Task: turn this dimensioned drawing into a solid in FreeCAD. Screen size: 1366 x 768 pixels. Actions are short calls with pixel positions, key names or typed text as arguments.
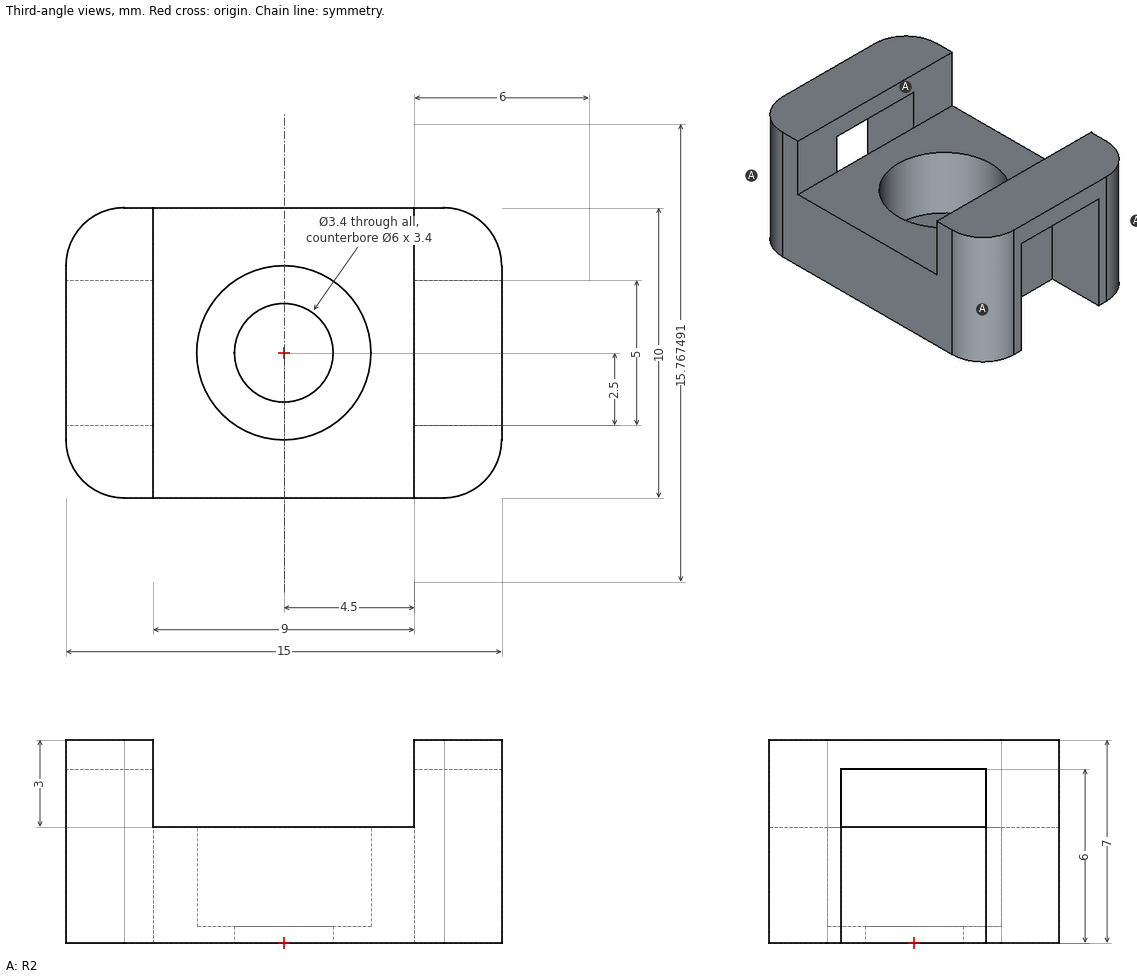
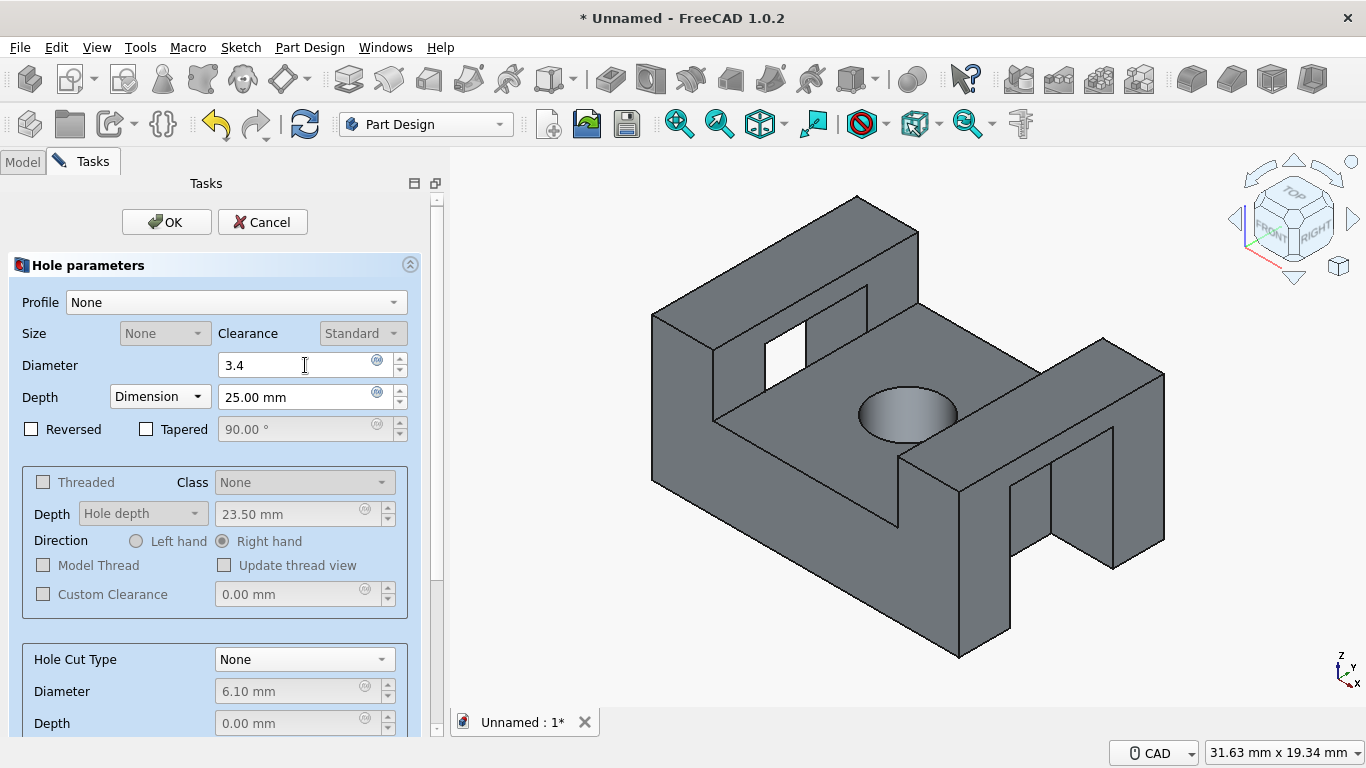
click(161, 396)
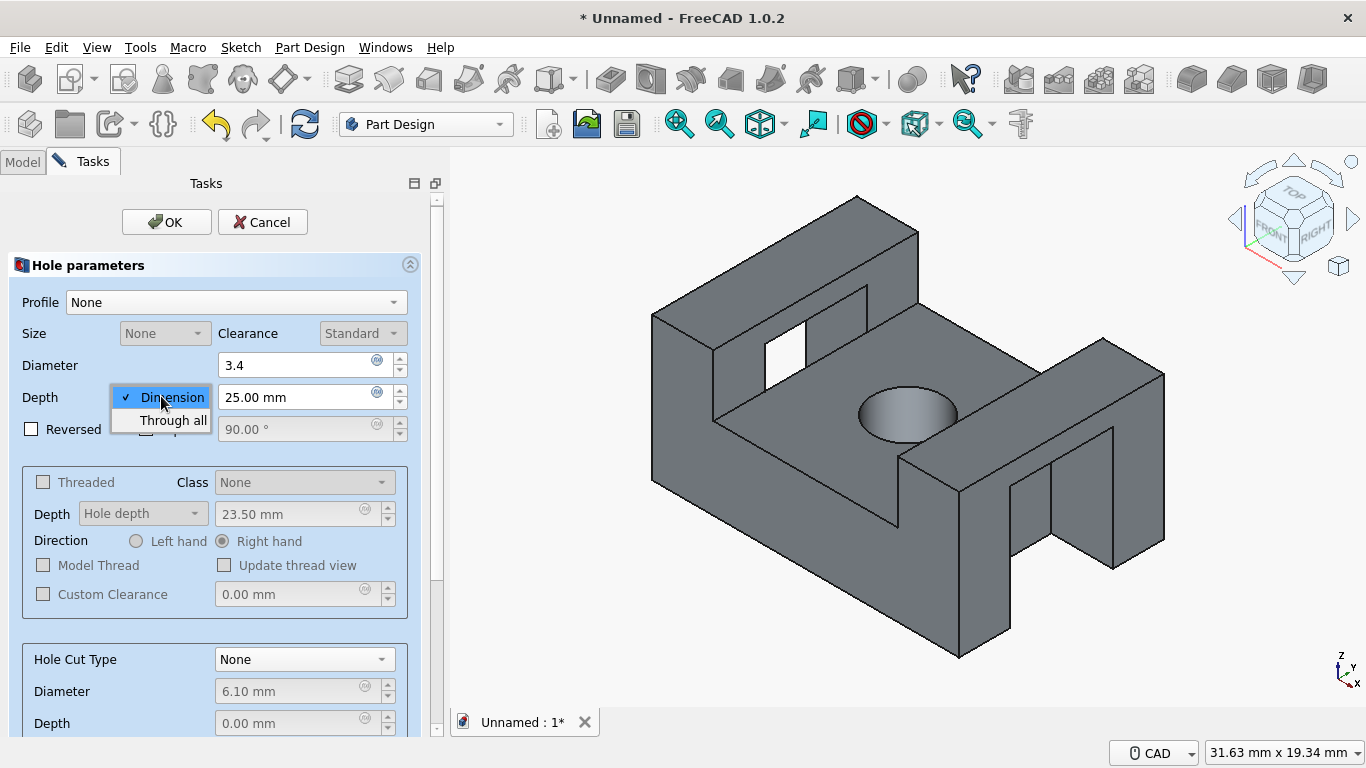
click(160, 420)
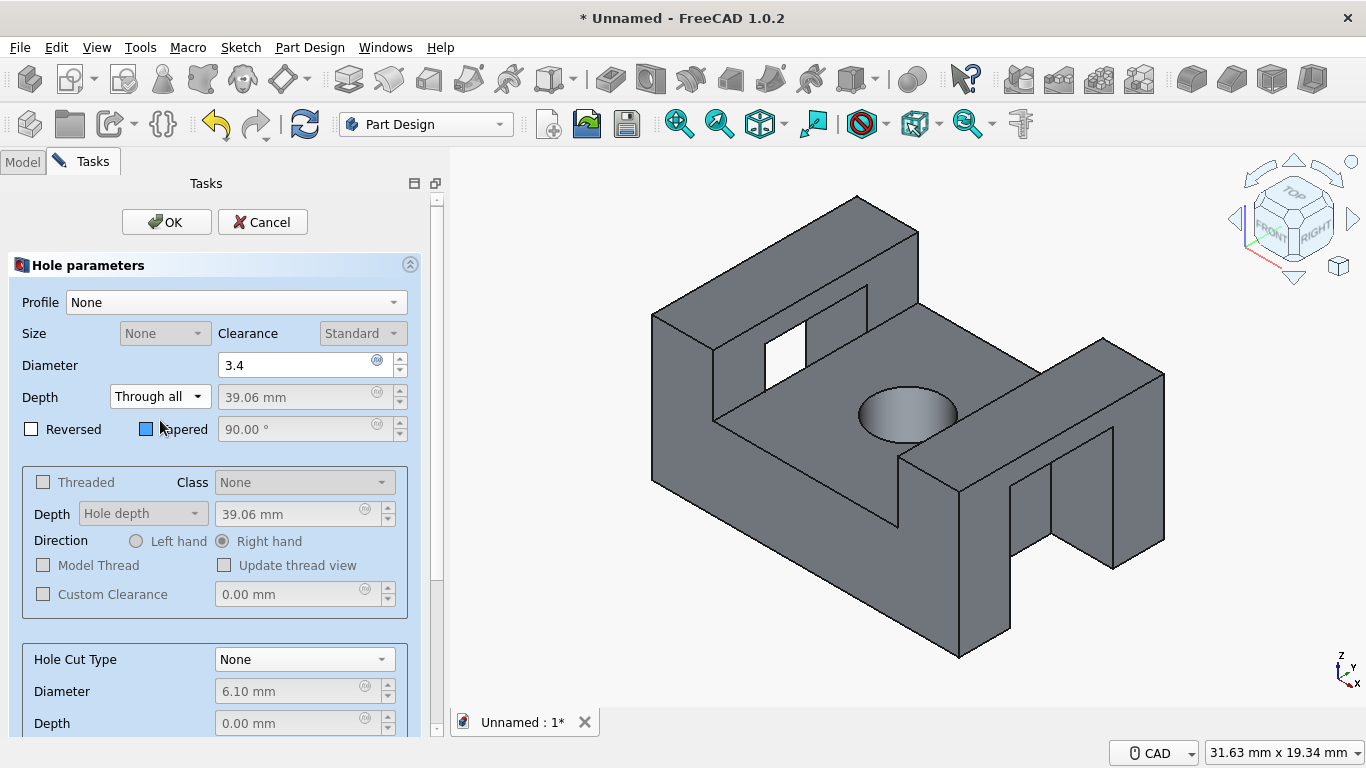
click(306, 660)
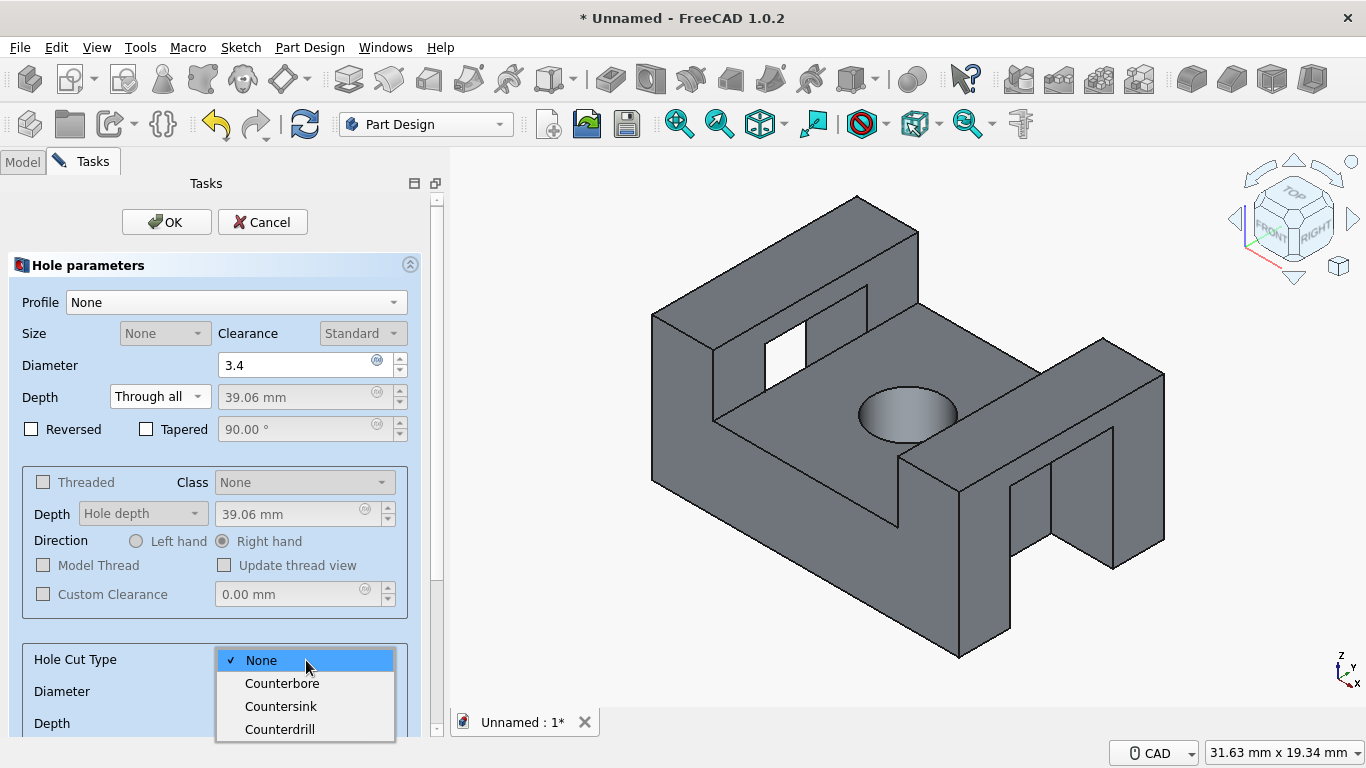
click(304, 684)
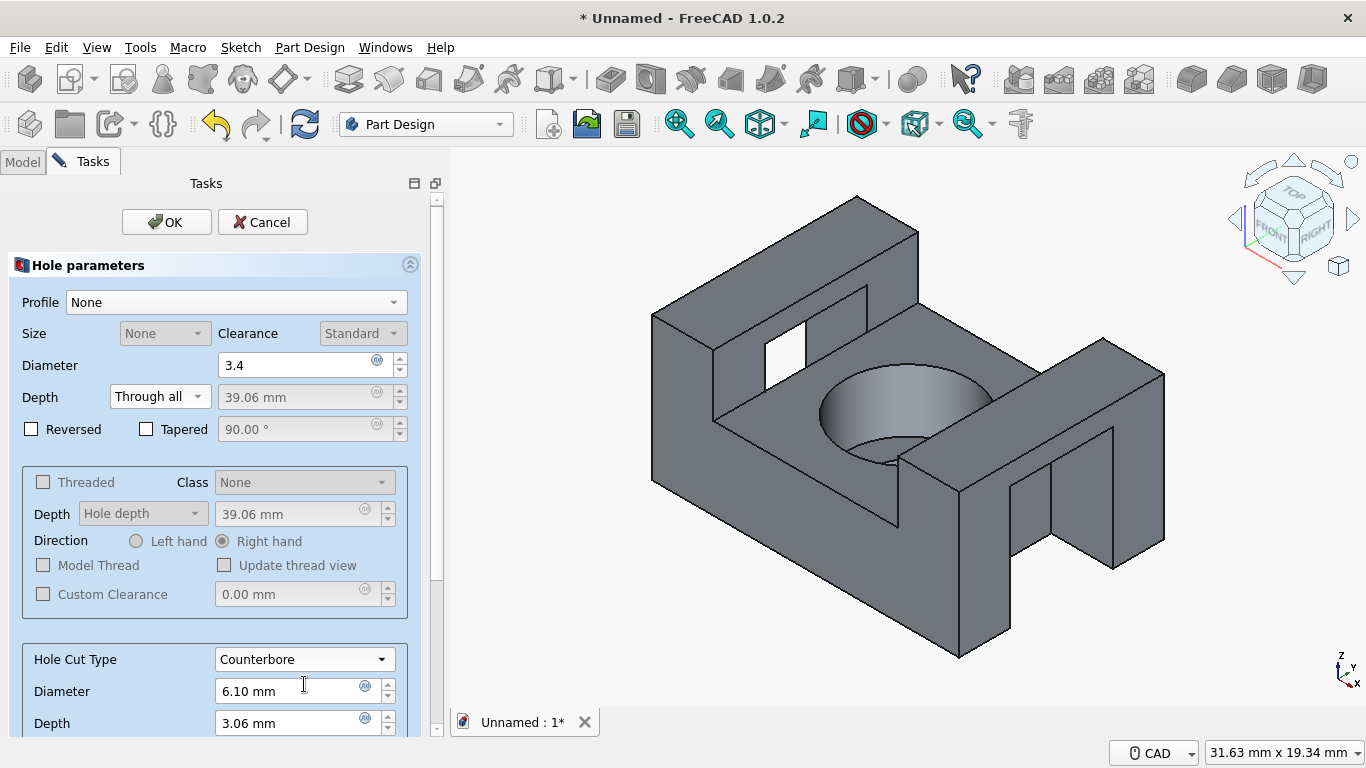
triple_click(298, 691)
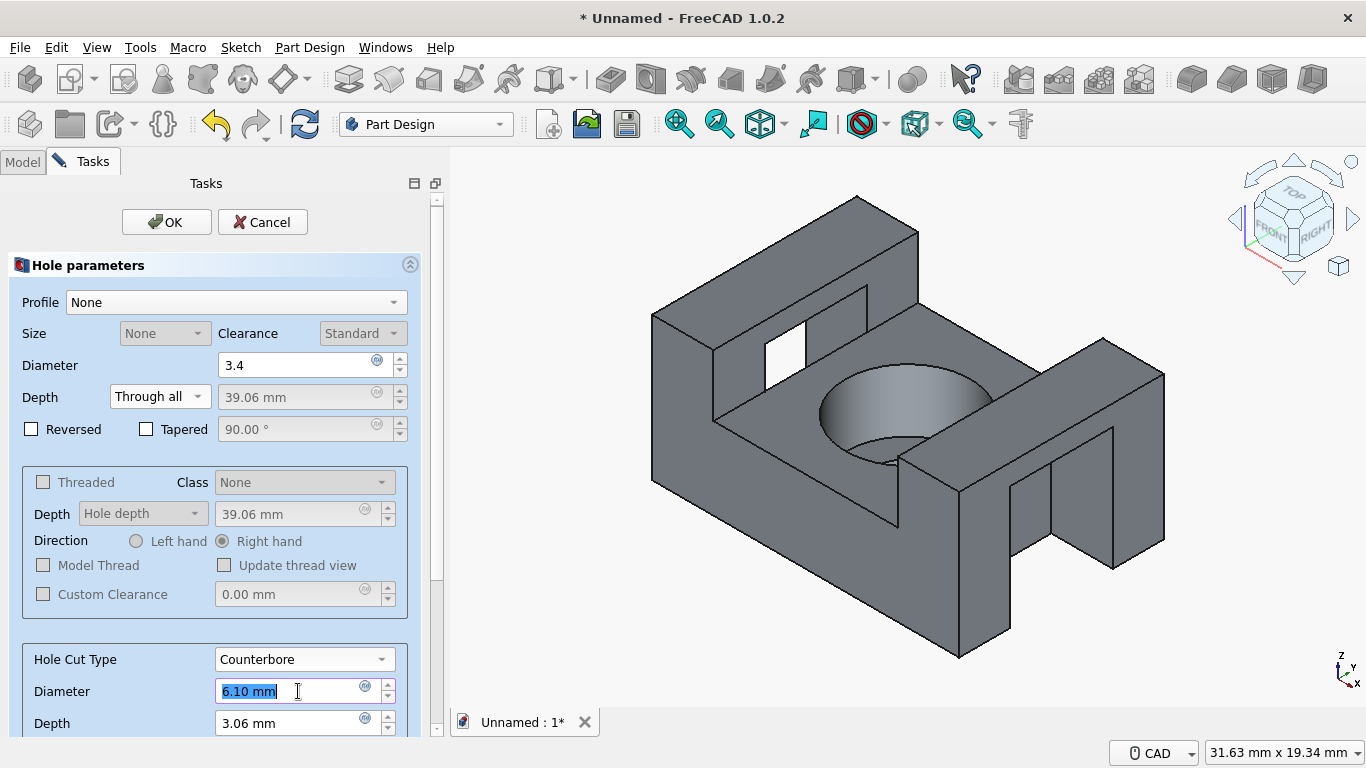
text(6)
key(Tab)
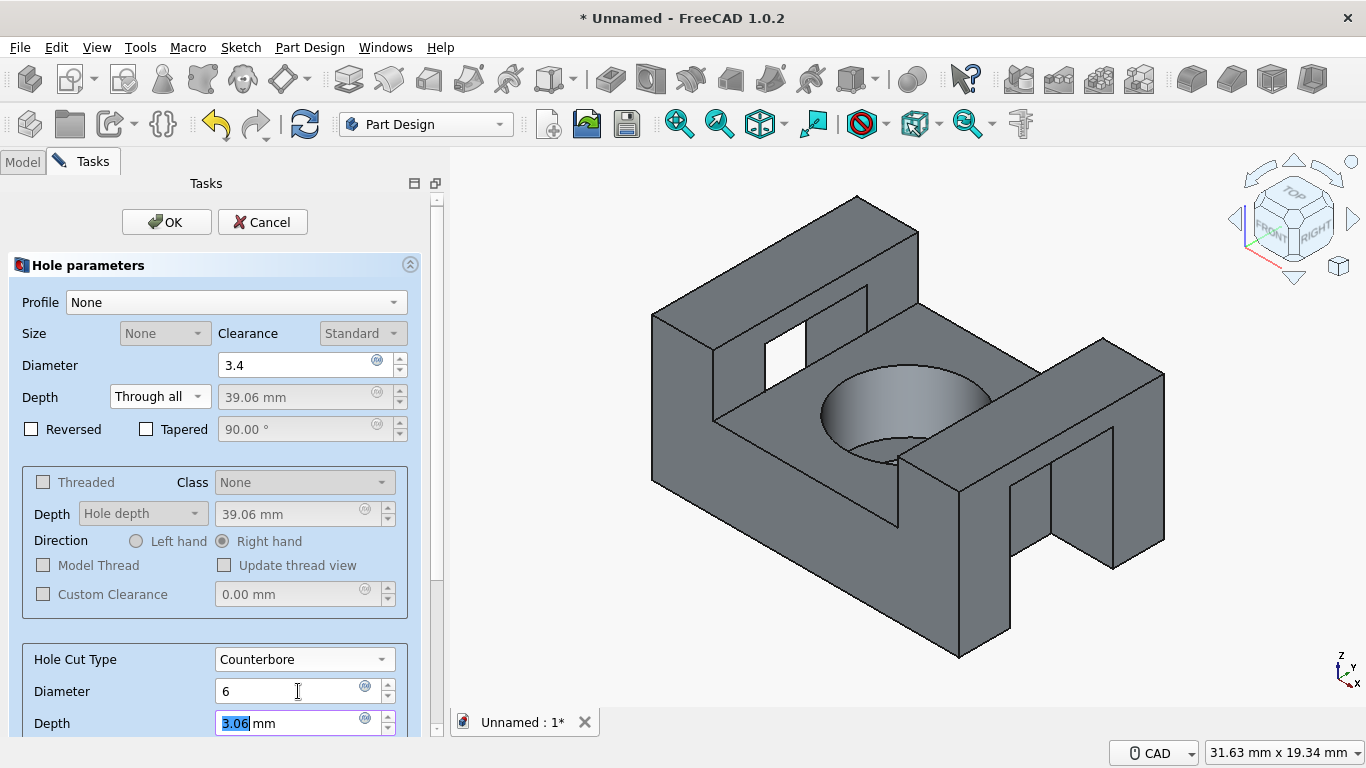
text(3.4)
key(Tab)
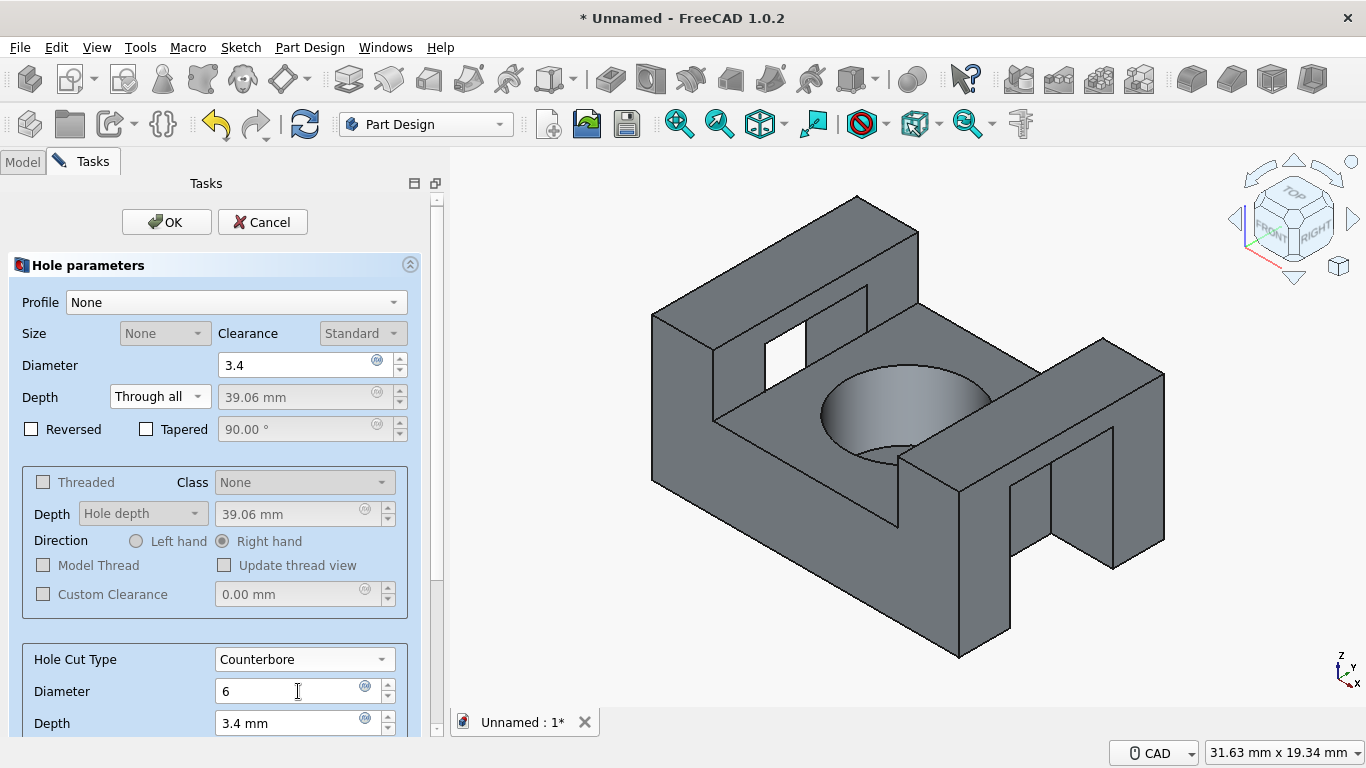
click(167, 222)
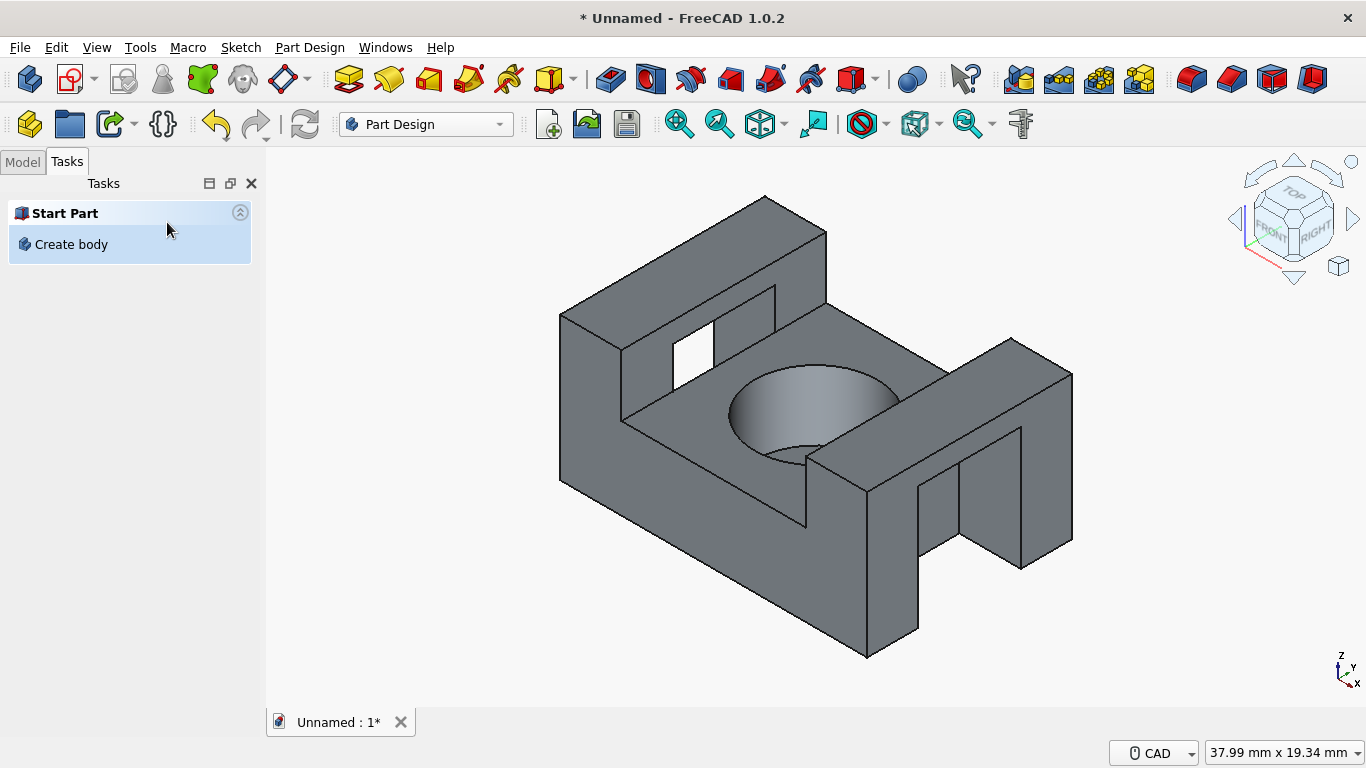
click(867, 574)